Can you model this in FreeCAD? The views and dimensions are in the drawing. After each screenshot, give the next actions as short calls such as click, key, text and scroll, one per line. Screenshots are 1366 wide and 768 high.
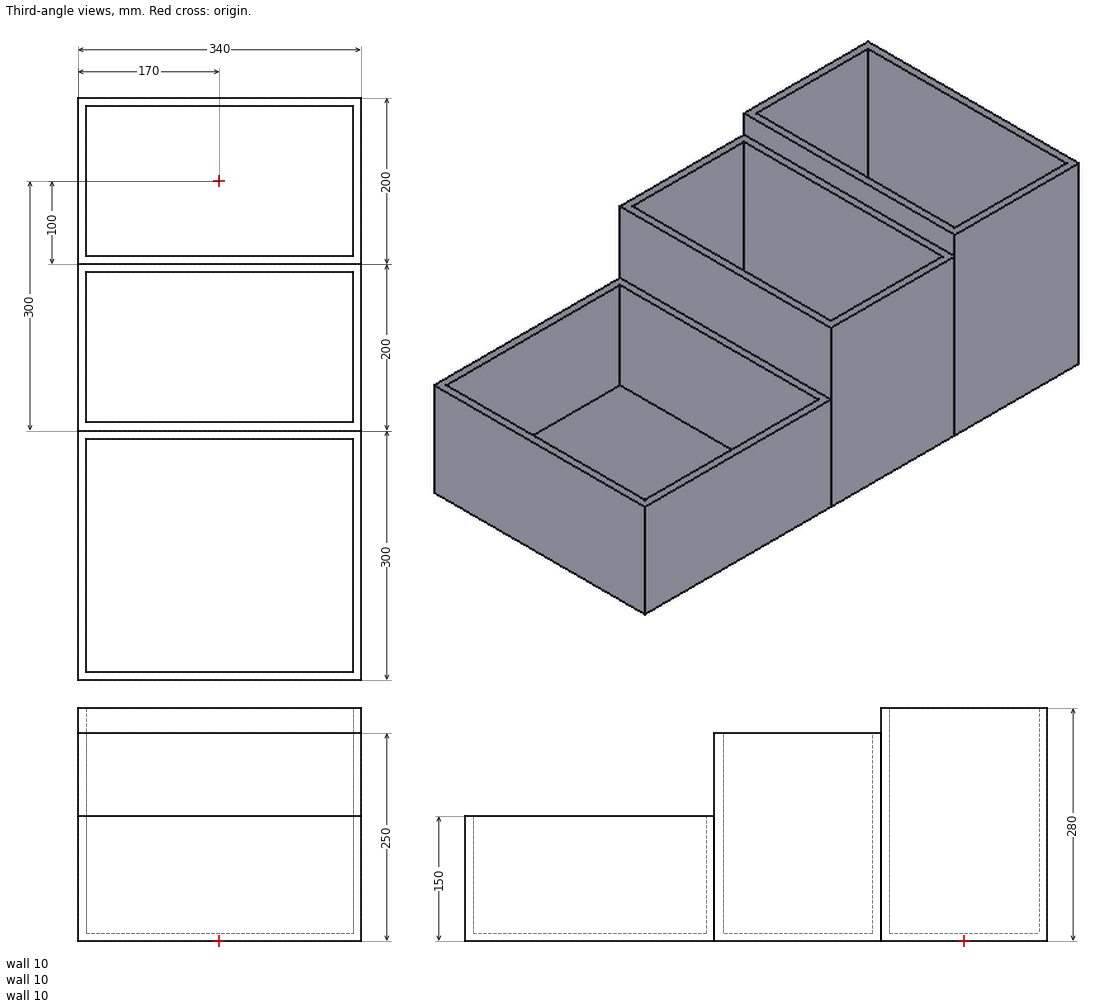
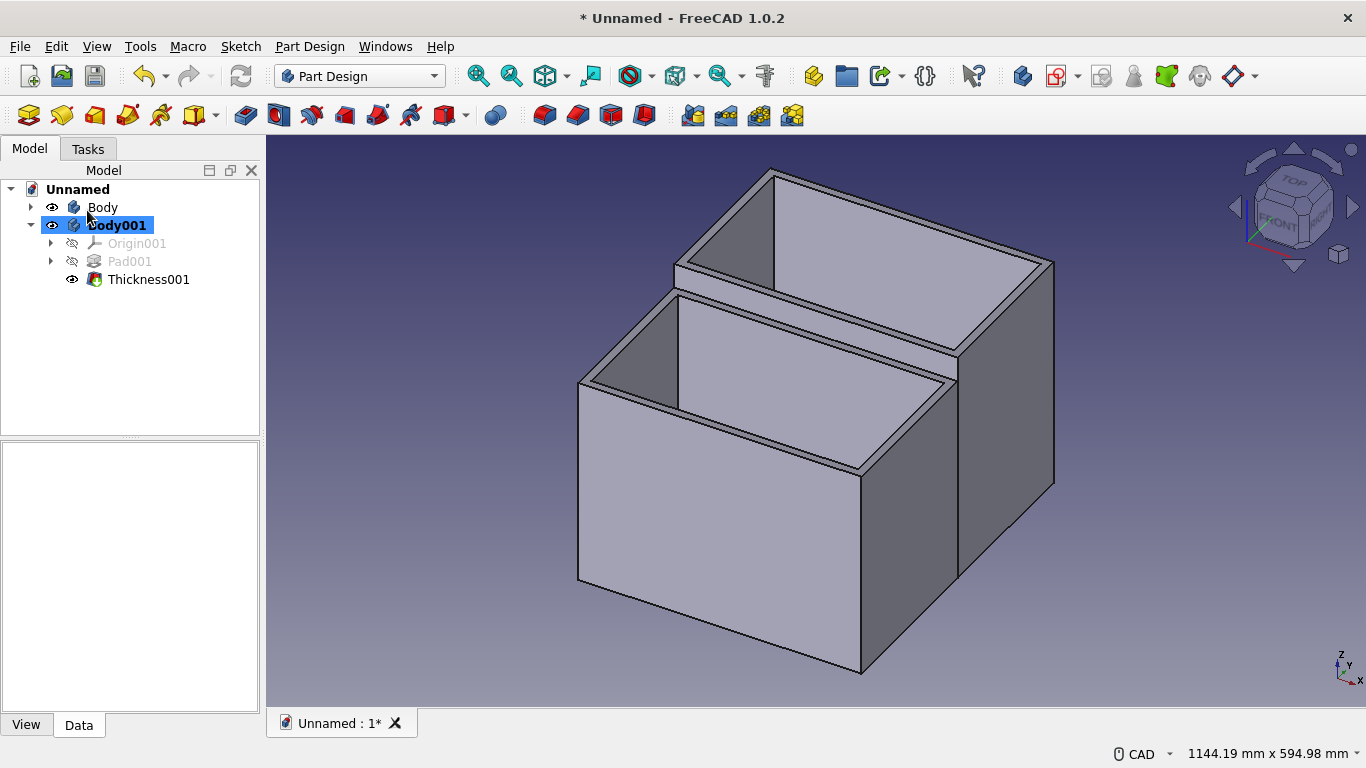
click(1023, 76)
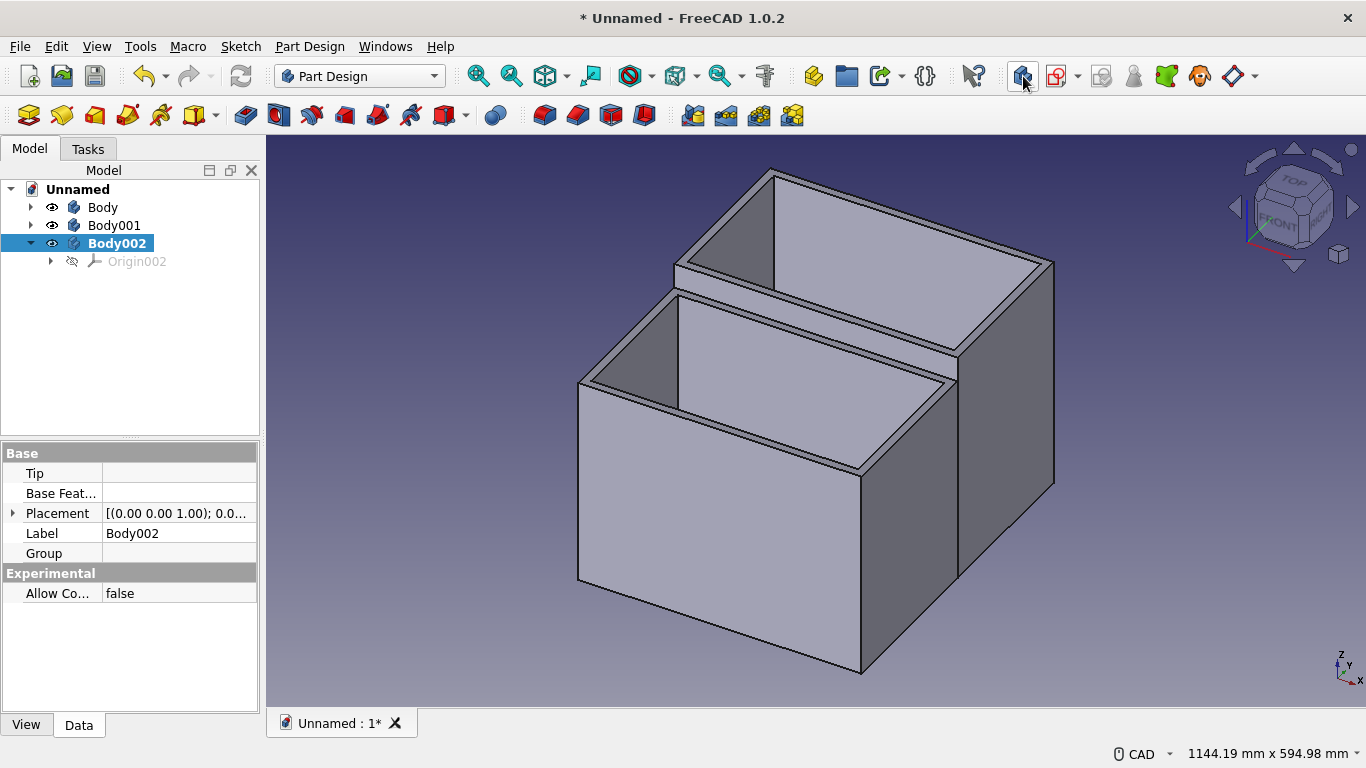
click(306, 667)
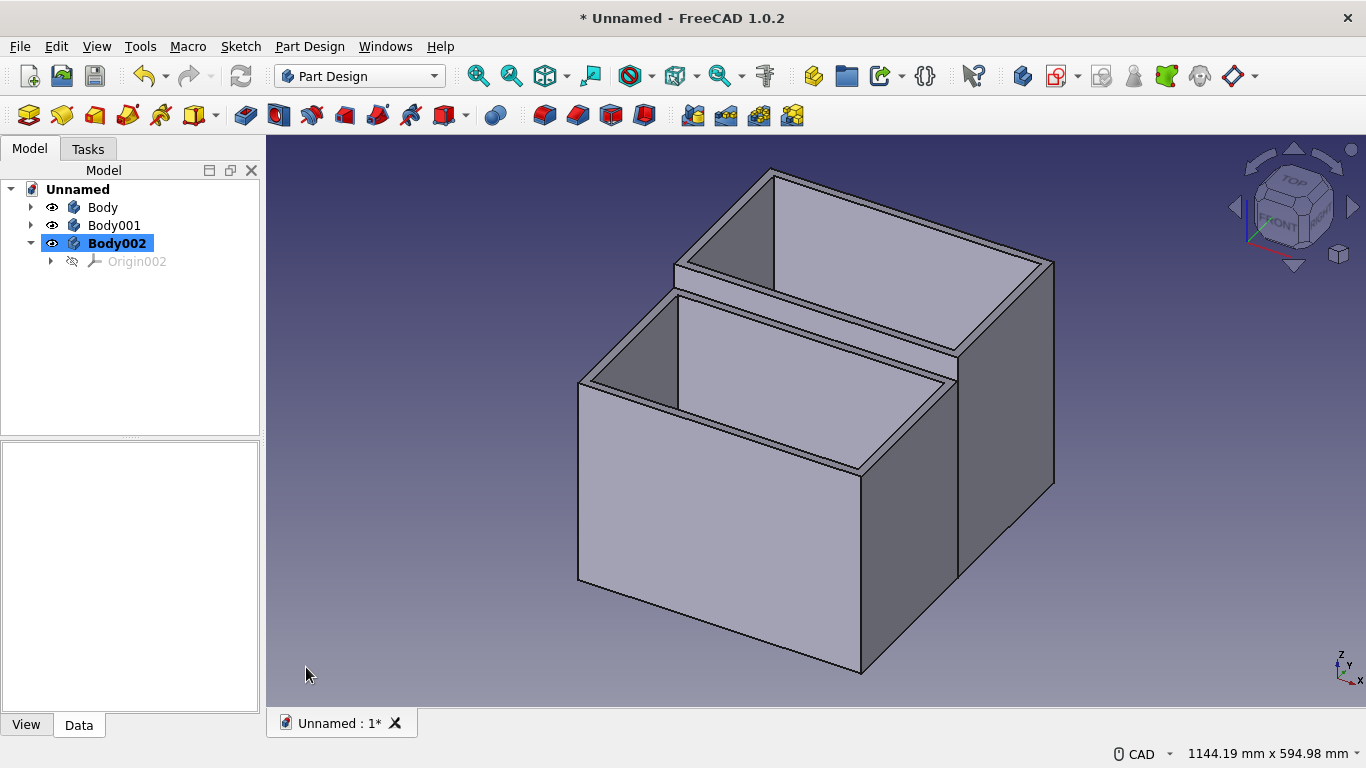
click(1056, 76)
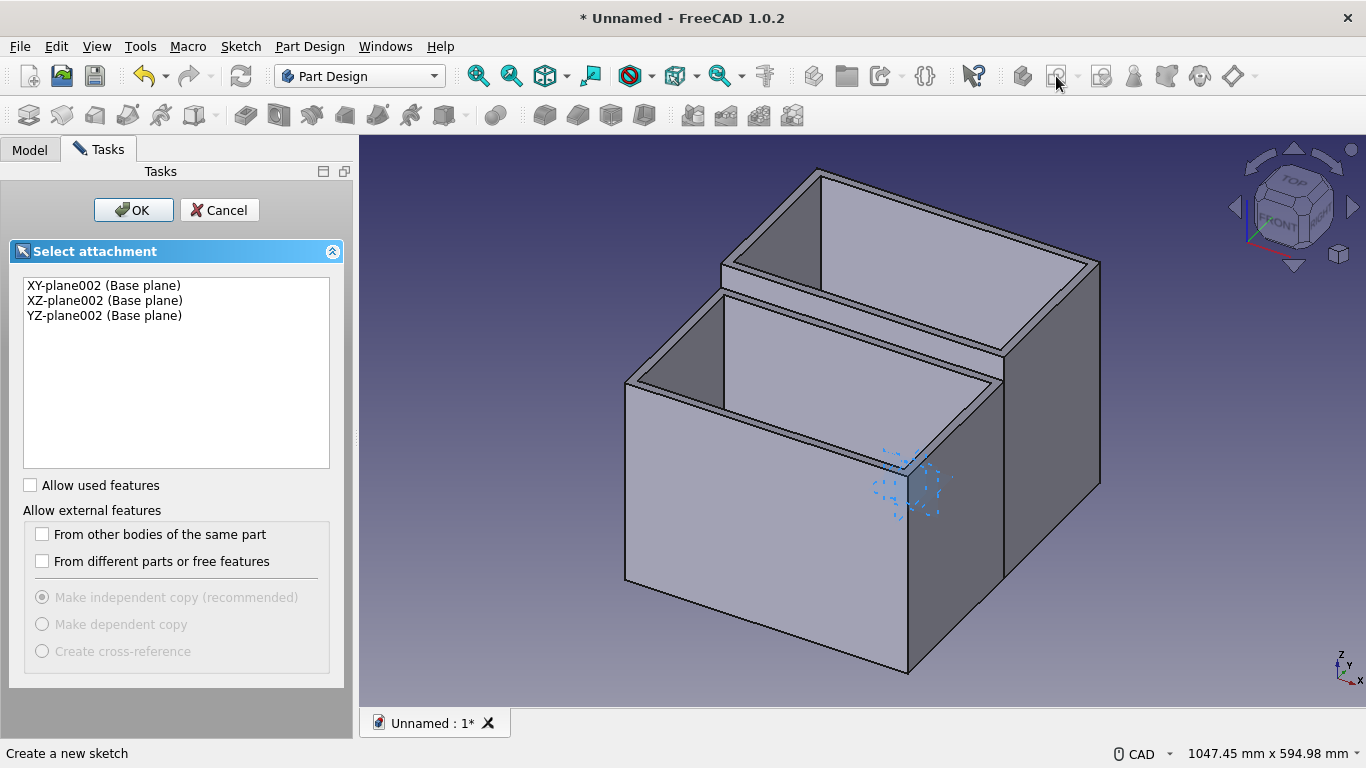
click(84, 286)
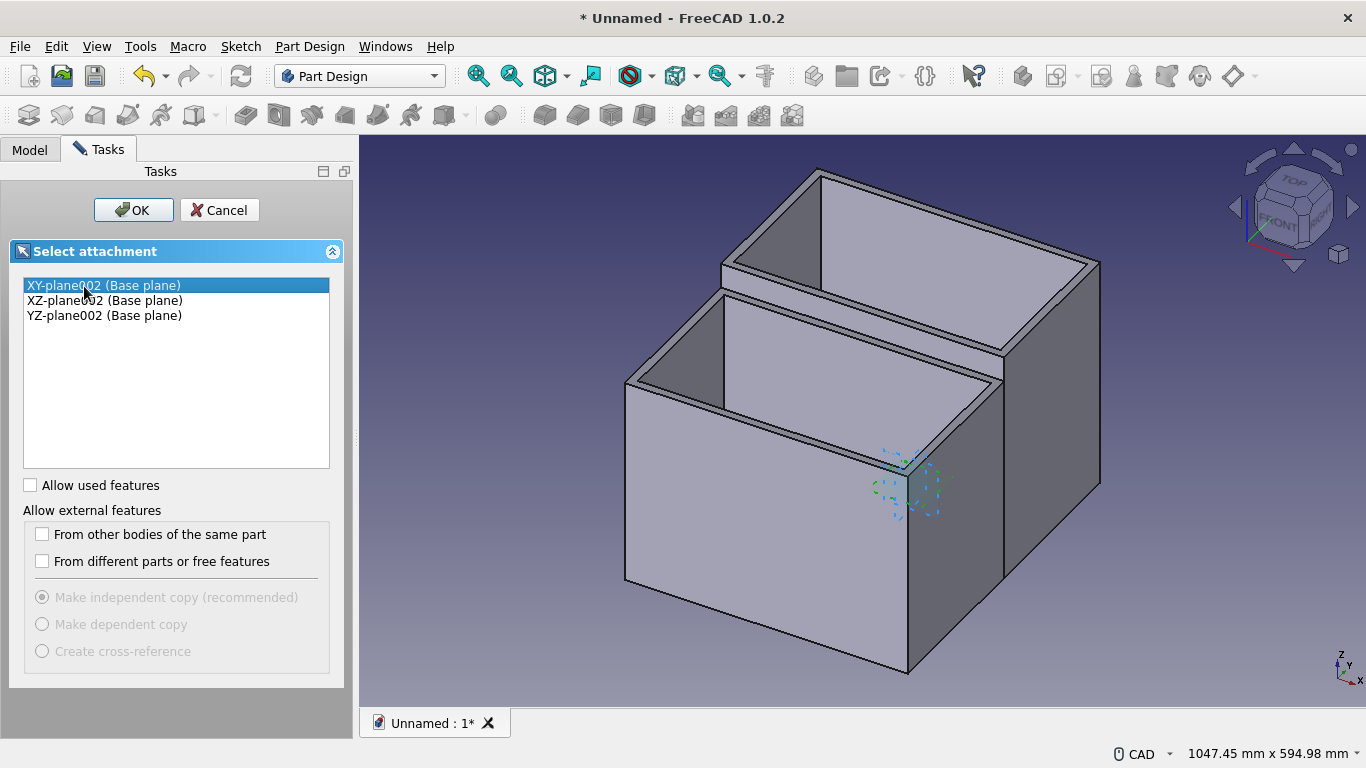
click(134, 210)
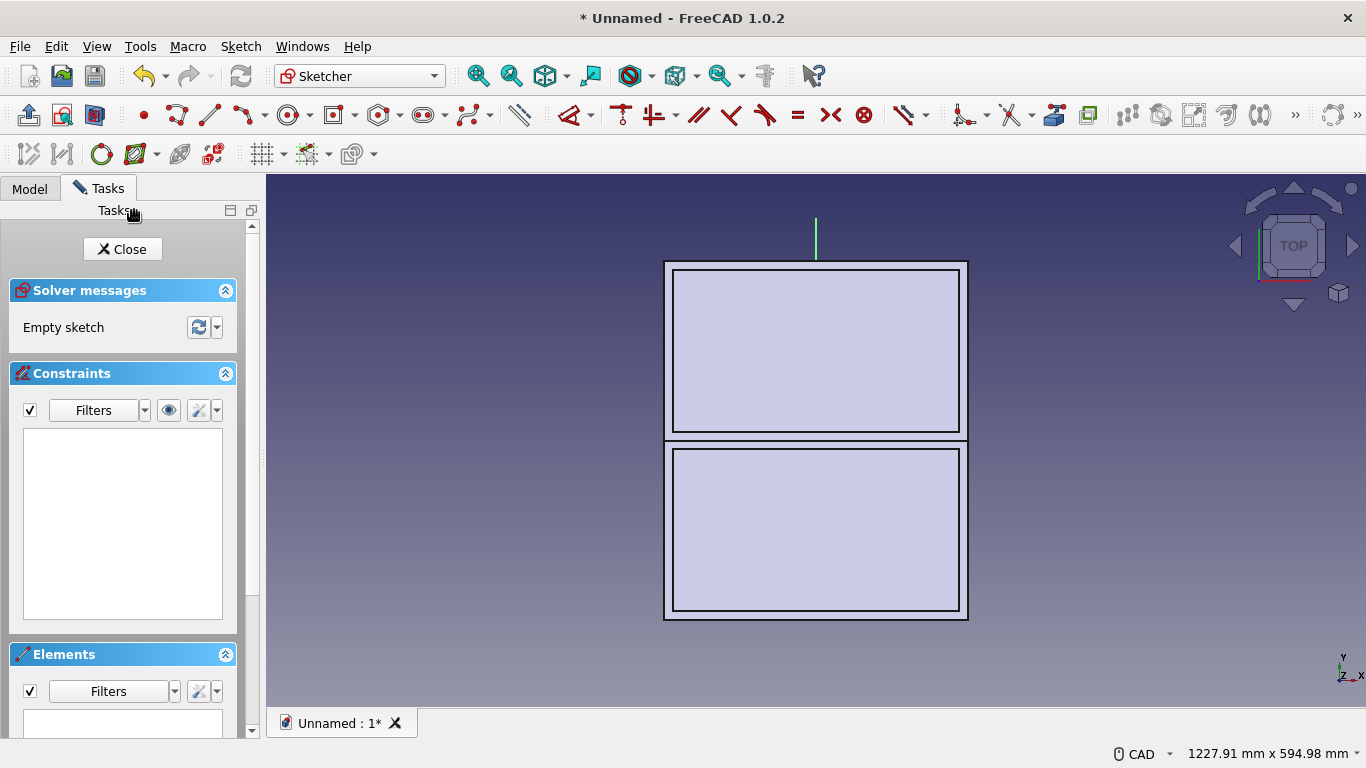
scroll(664, 223, down, 3)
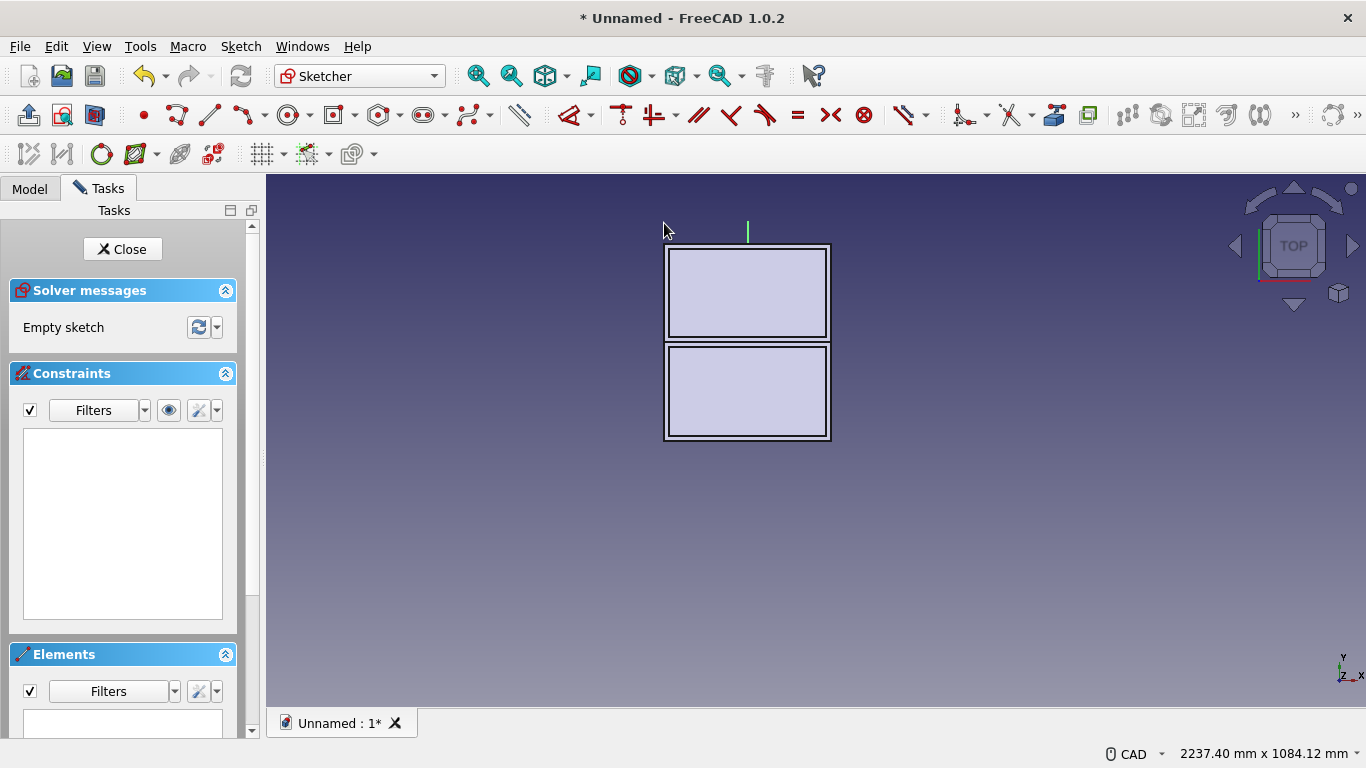
key(g)
key(r)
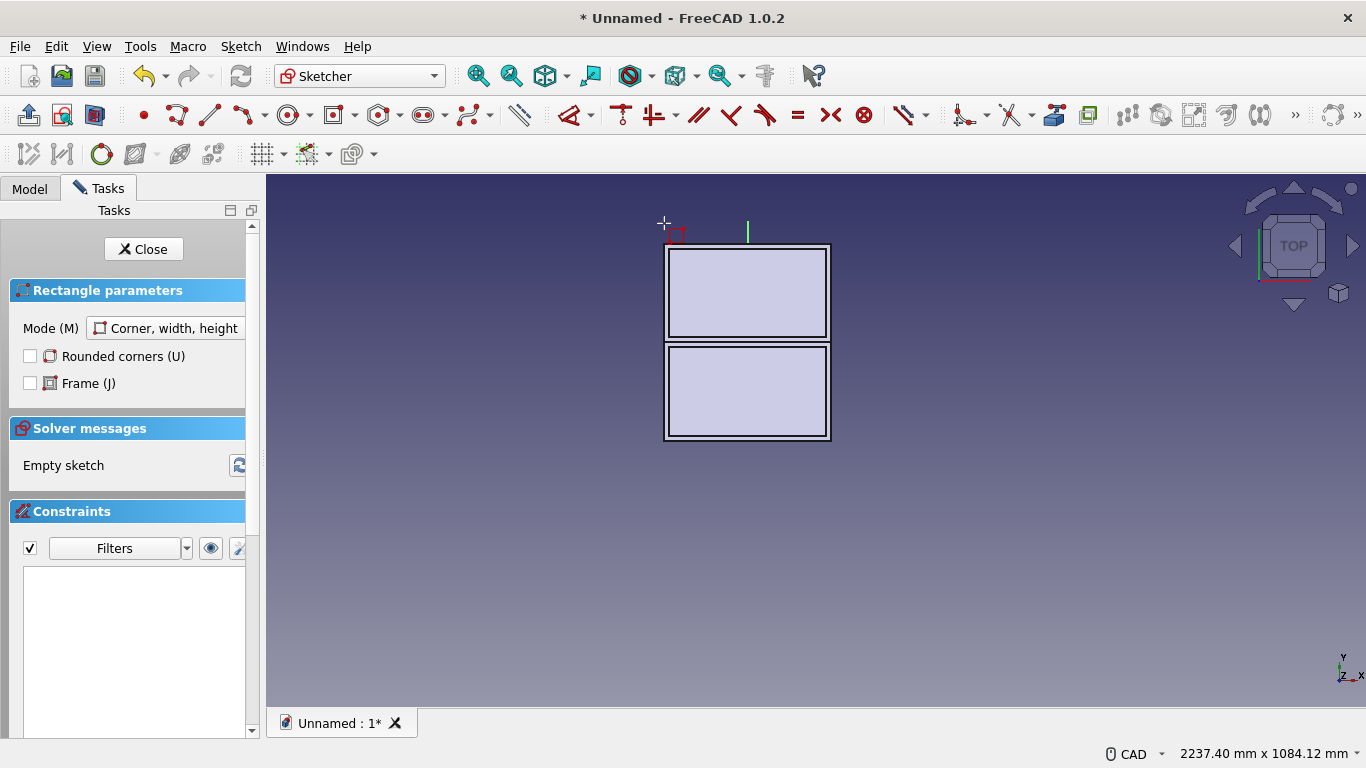
click(664, 441)
move(831, 588)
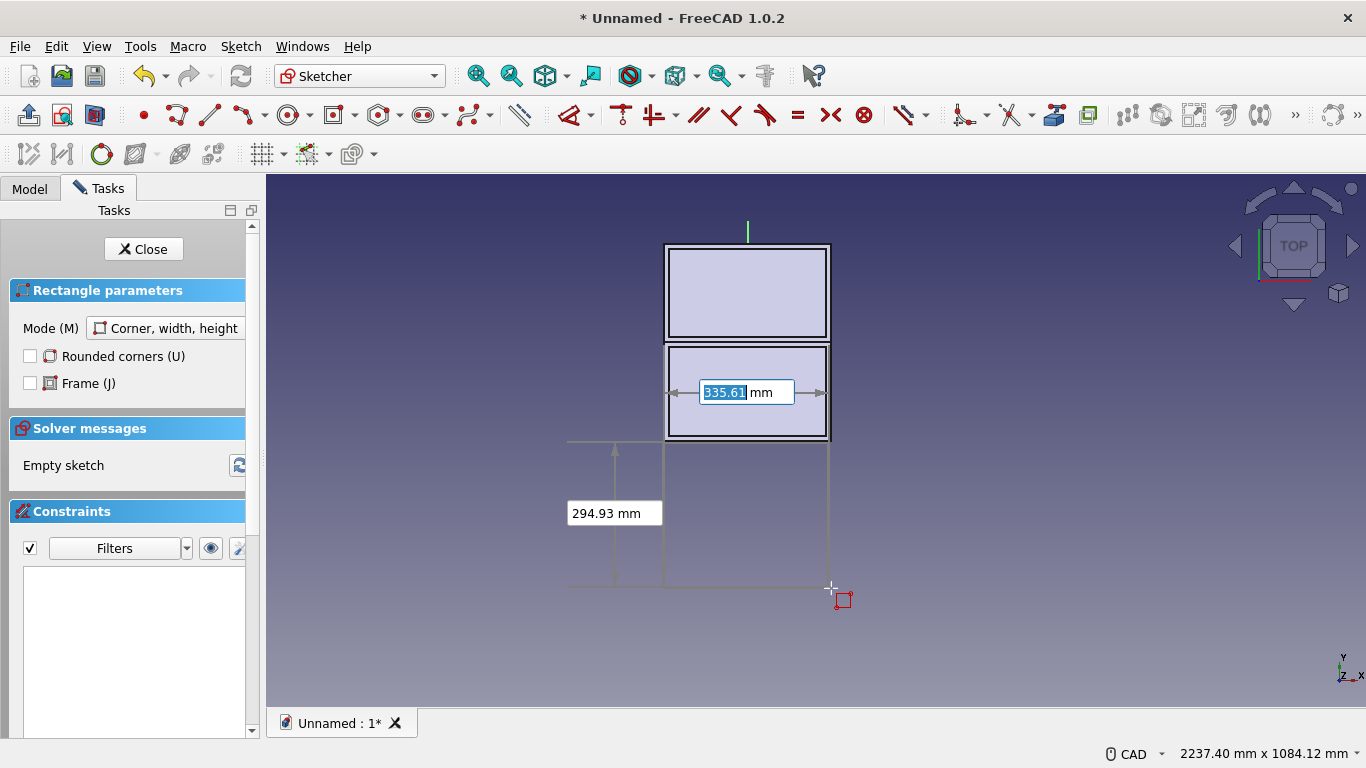
text(340)
key(Tab)
text(300)
key(Return)
key(Escape)